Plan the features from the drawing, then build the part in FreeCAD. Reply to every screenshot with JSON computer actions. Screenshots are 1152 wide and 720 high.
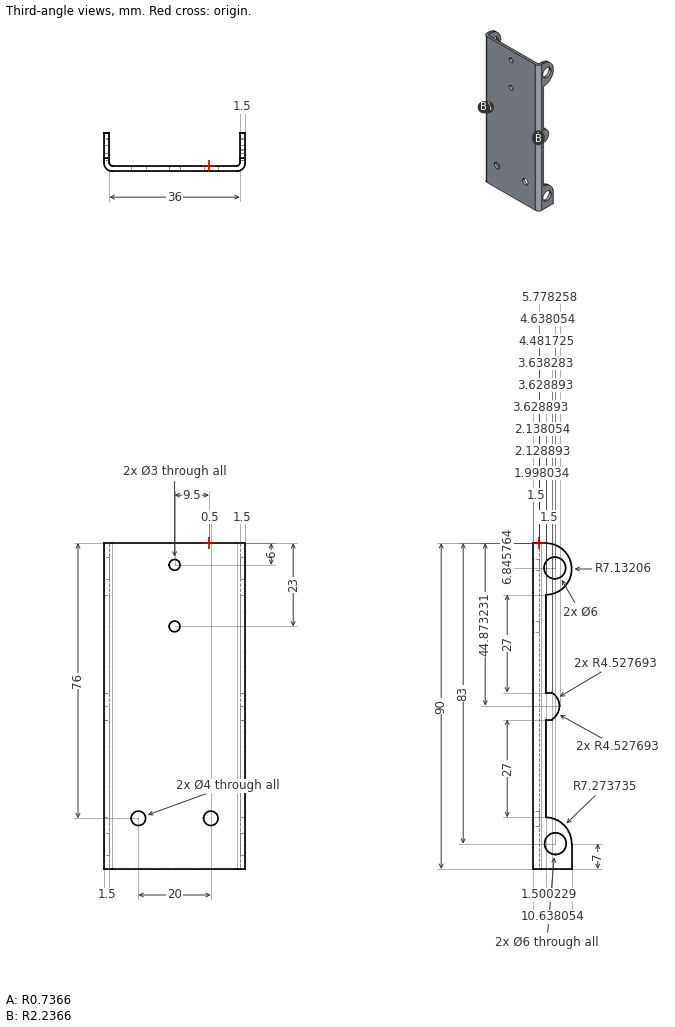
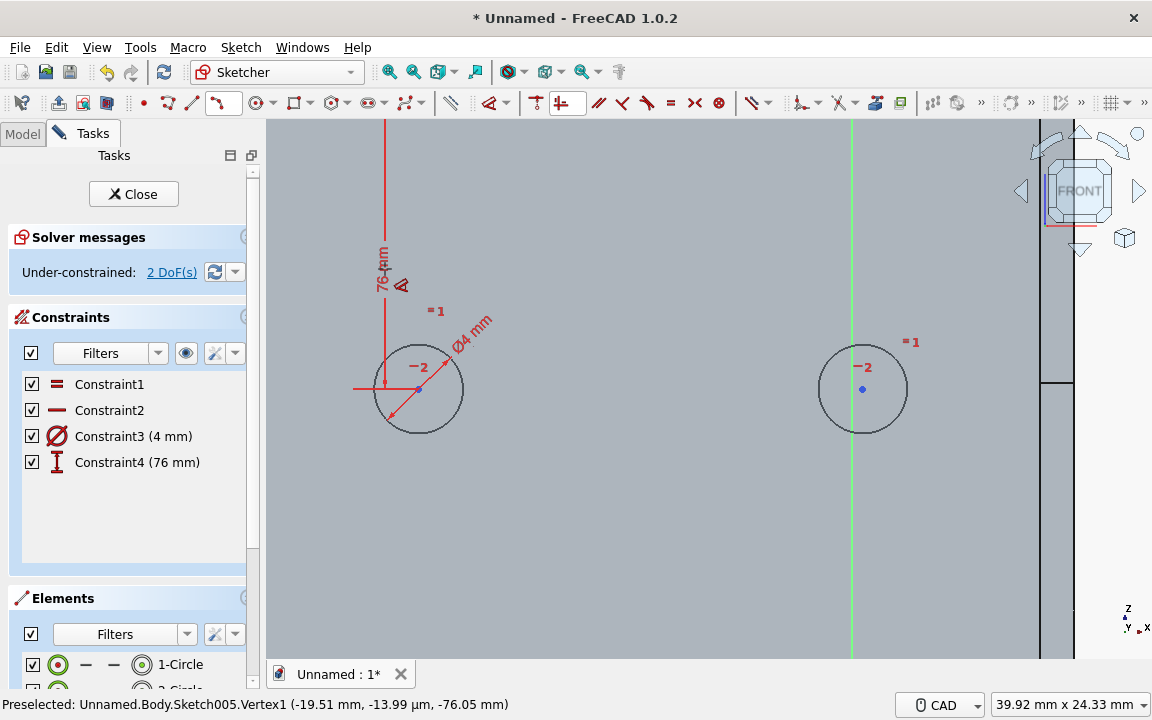
{"action": "scroll", "coordinate": [863, 389], "scroll_direction": "up", "scroll_amount": 7}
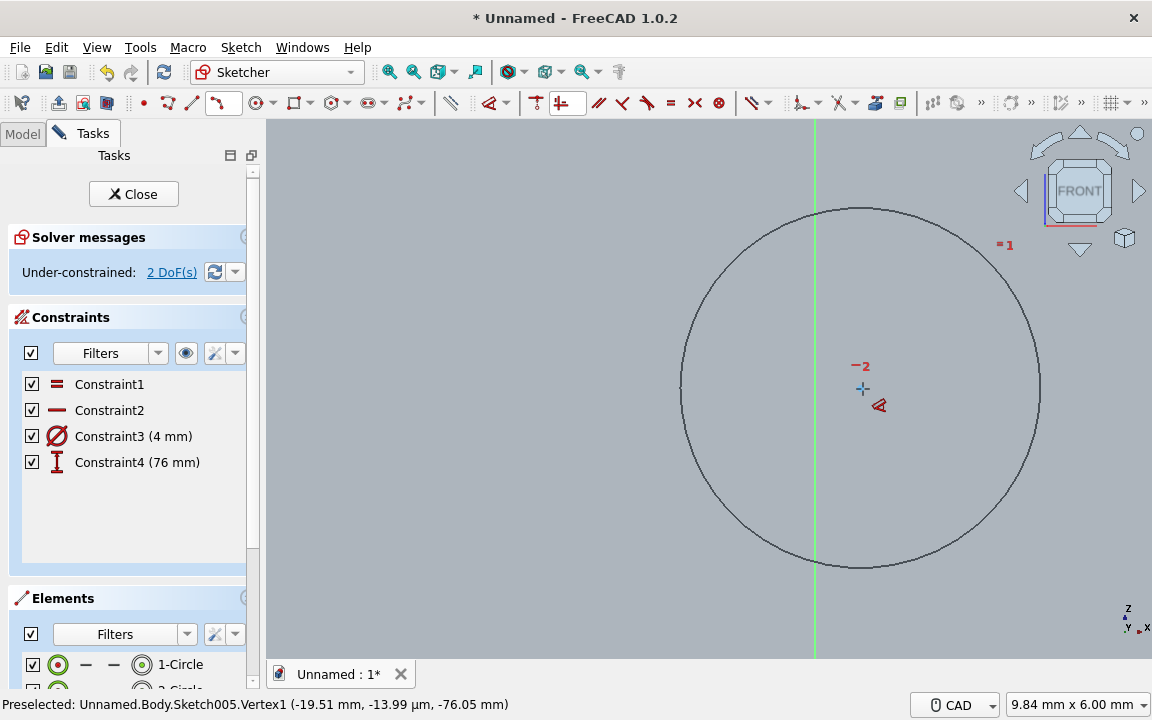
{"action": "left_click", "coordinate": [860, 388]}
{"action": "left_click", "coordinate": [838, 422]}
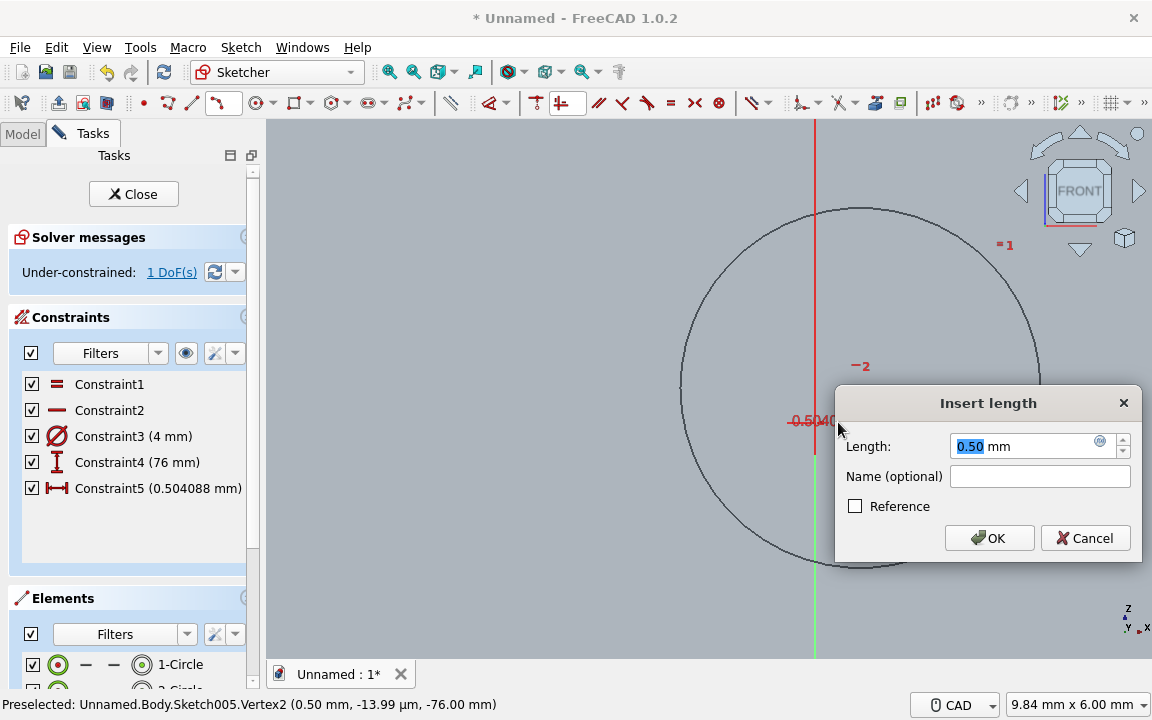
{"action": "type", "text": "0.5"}
{"action": "key", "text": "Return"}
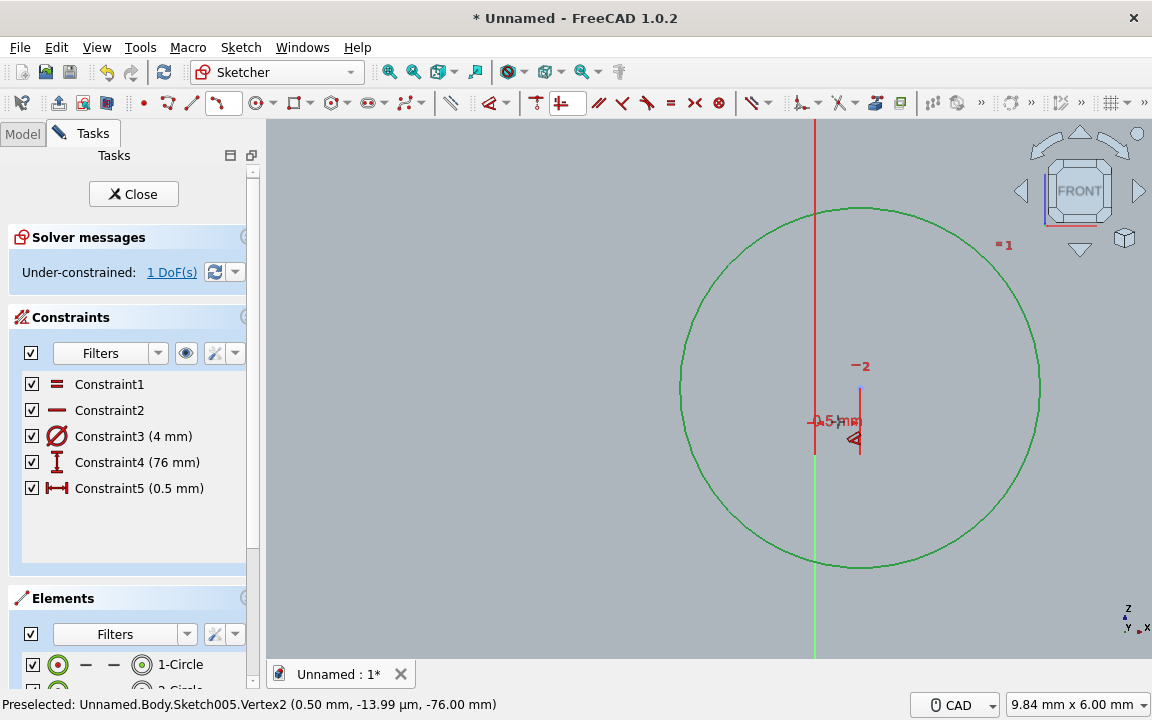
{"action": "scroll", "coordinate": [863, 389], "scroll_direction": "down", "scroll_amount": 7}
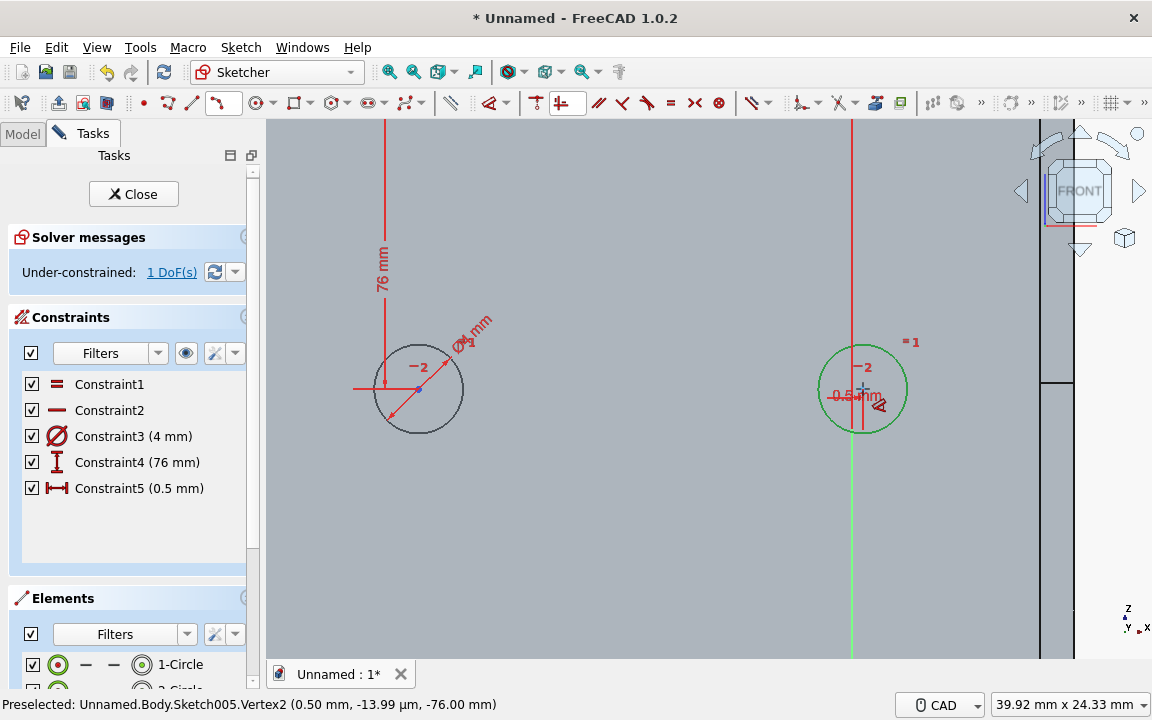
{"action": "left_click", "coordinate": [419, 389]}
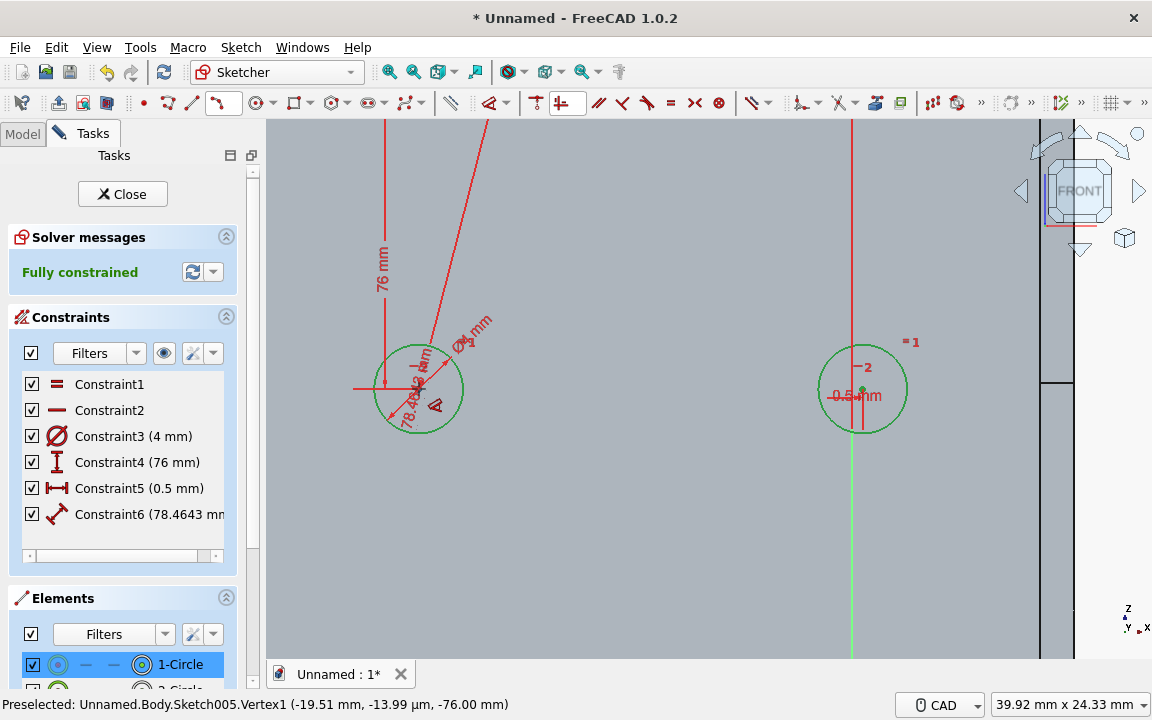
{"action": "left_click", "coordinate": [863, 389]}
{"action": "left_click", "coordinate": [641, 423]}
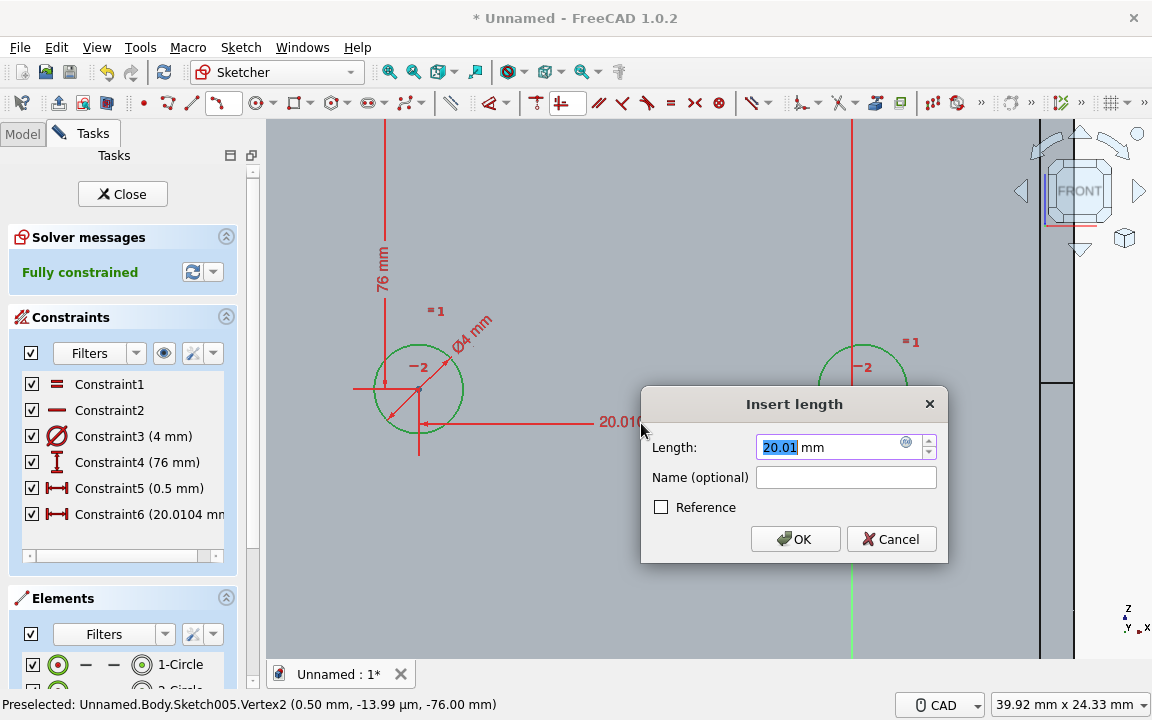
{"action": "type", "text": "20"}
{"action": "key", "text": "Return"}
{"action": "key", "text": "Escape"}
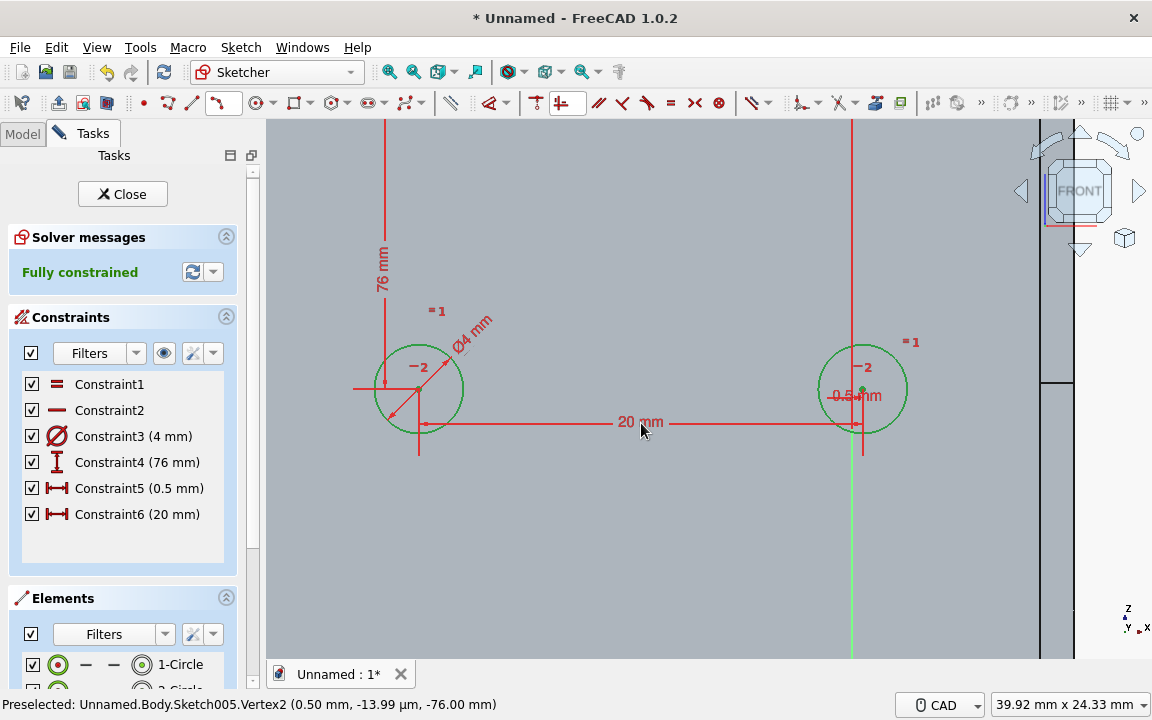
{"action": "left_click", "coordinate": [123, 194]}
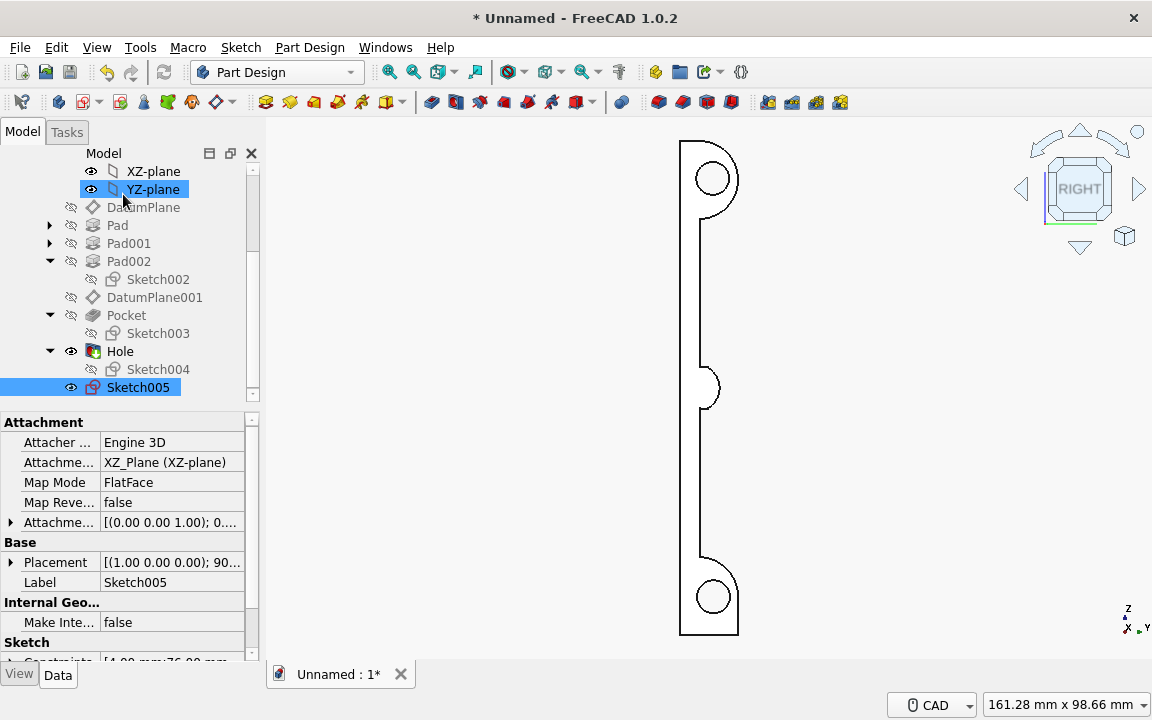
{"action": "left_click", "coordinate": [456, 102]}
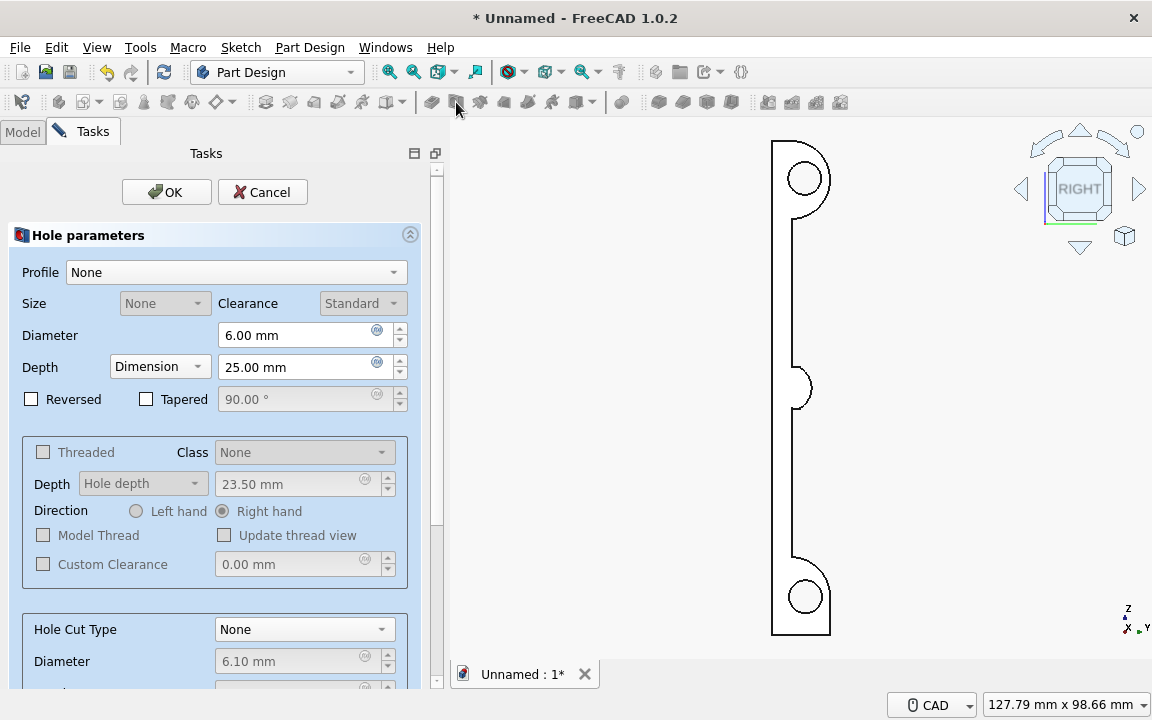
{"action": "triple_click", "coordinate": [305, 335]}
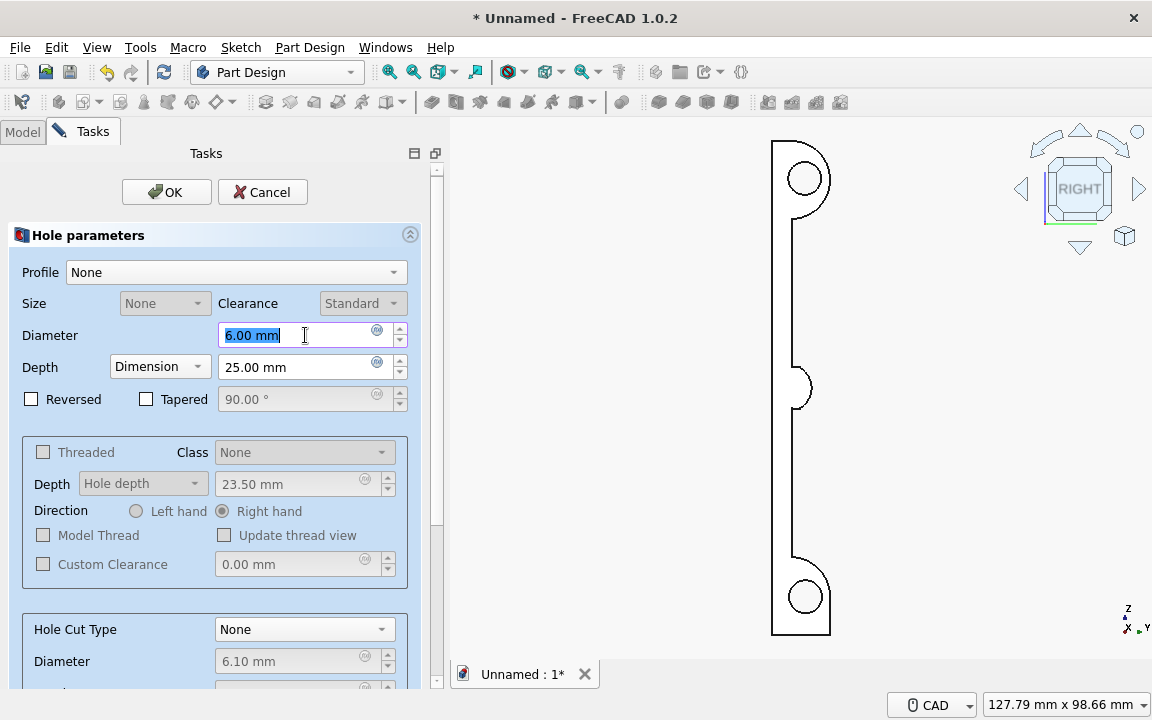
{"action": "type", "text": "4"}
{"action": "key", "text": "Tab"}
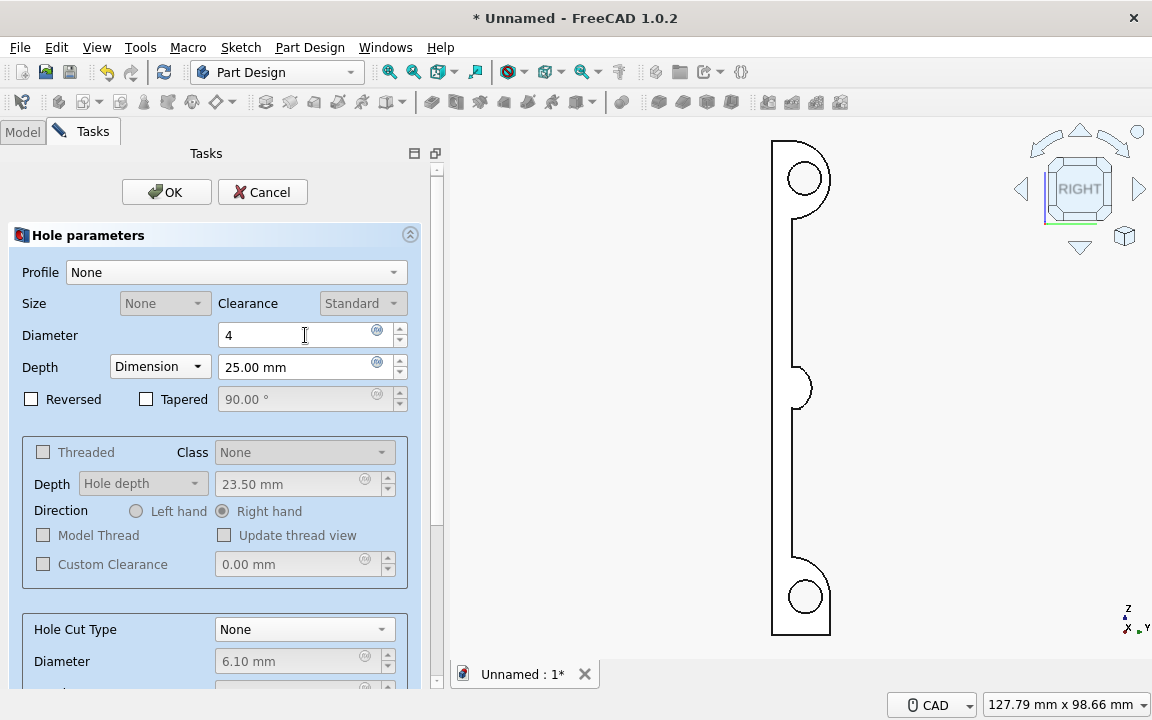
{"action": "left_click", "coordinate": [161, 366]}